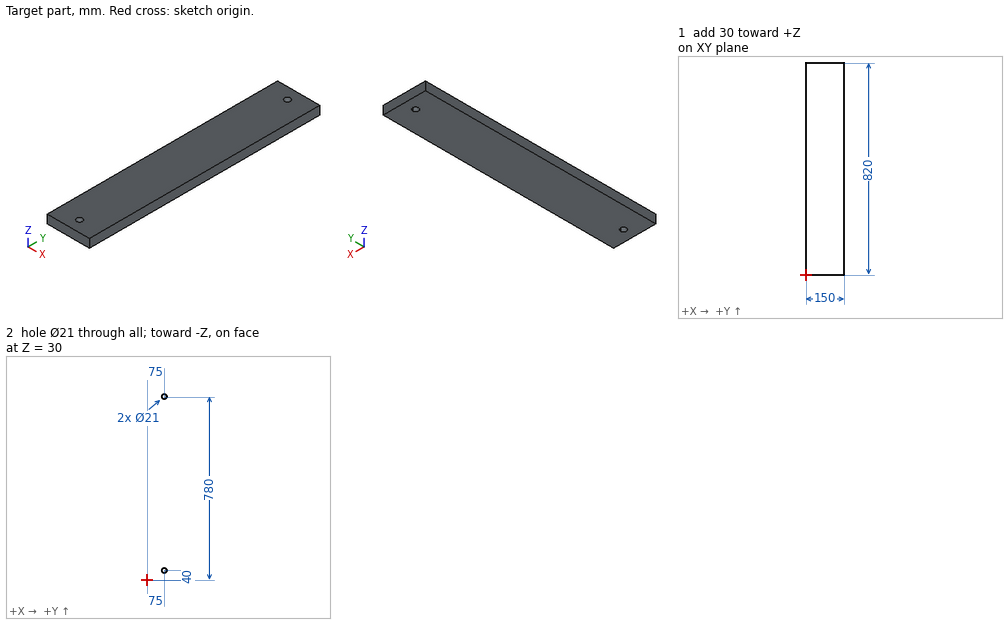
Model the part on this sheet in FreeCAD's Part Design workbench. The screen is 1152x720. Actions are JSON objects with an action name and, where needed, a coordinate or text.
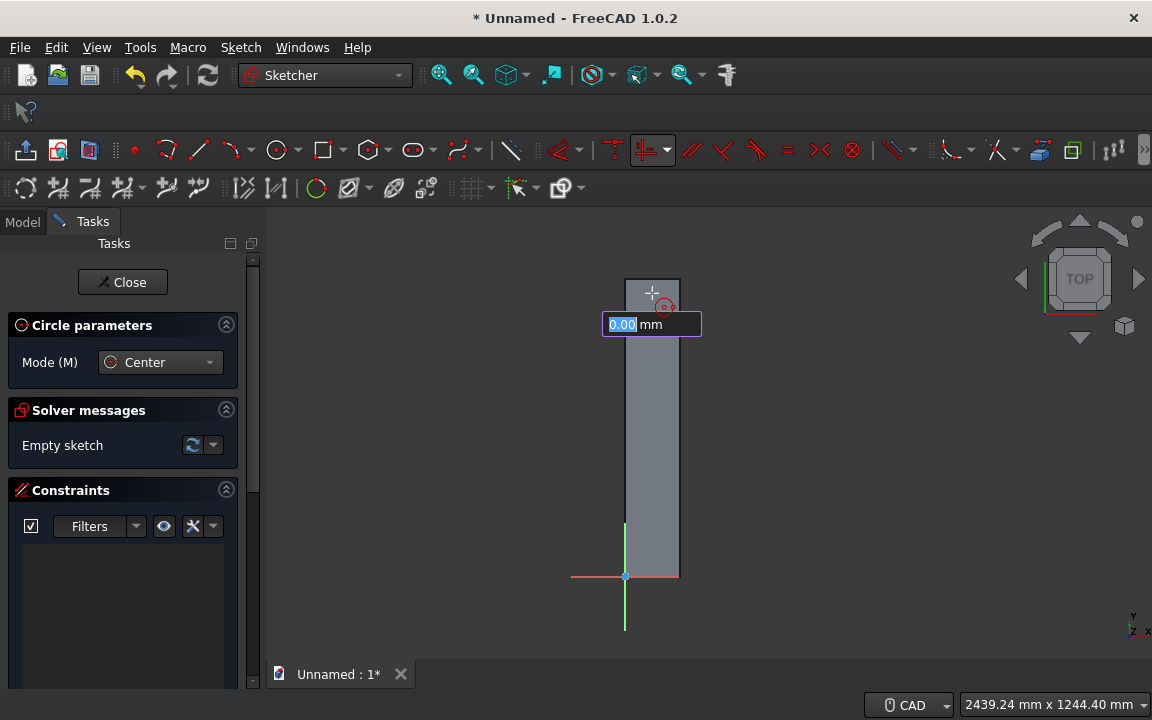
{"action": "scroll", "coordinate": [655, 291], "scroll_direction": "up", "scroll_amount": 8}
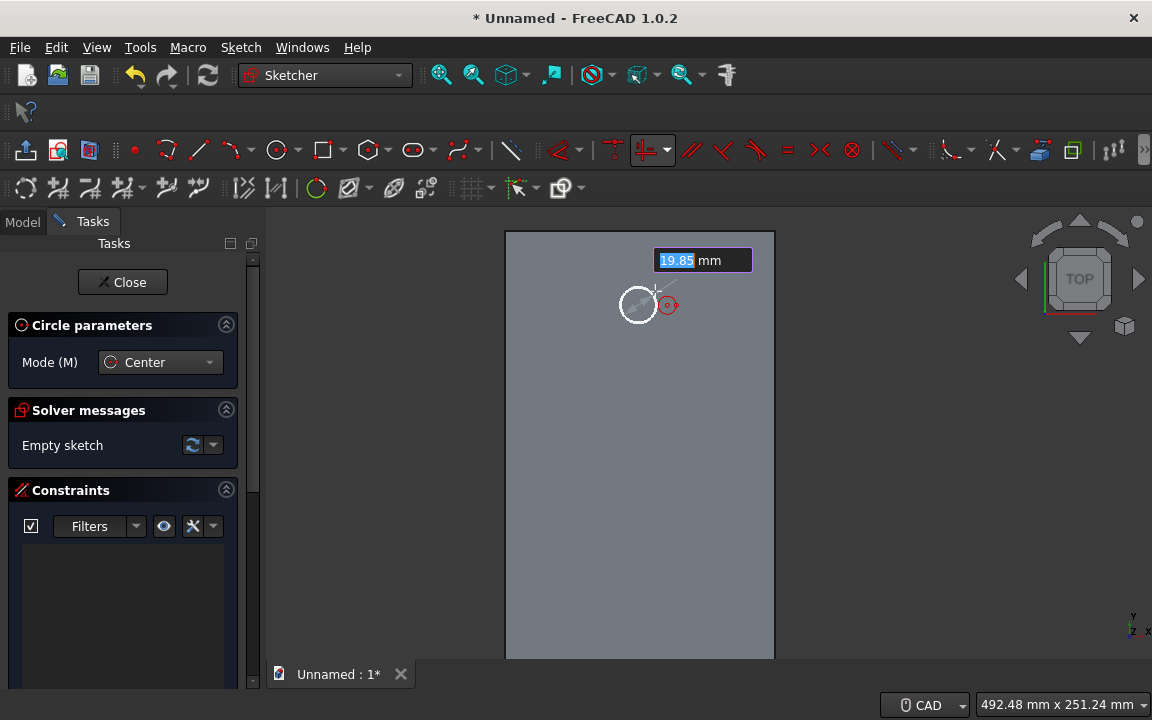
{"action": "left_click", "coordinate": [654, 289]}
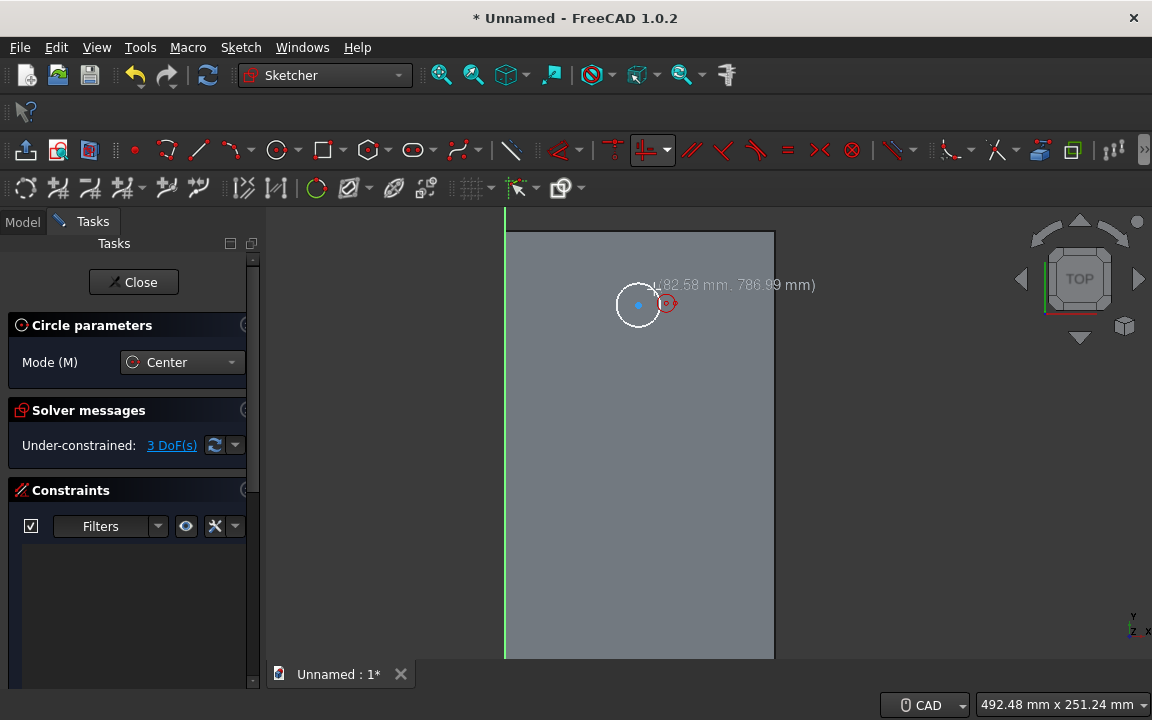
{"action": "scroll", "coordinate": [655, 291], "scroll_direction": "down", "scroll_amount": 8}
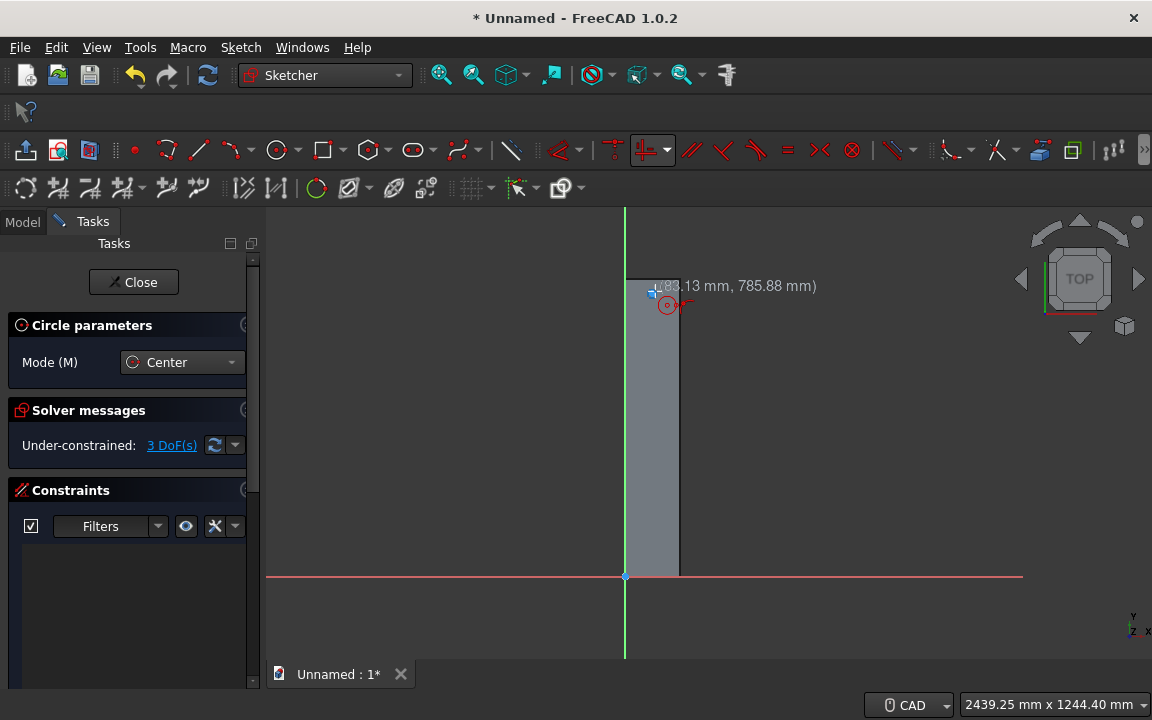
{"action": "scroll", "coordinate": [652, 562], "scroll_direction": "up", "scroll_amount": 9}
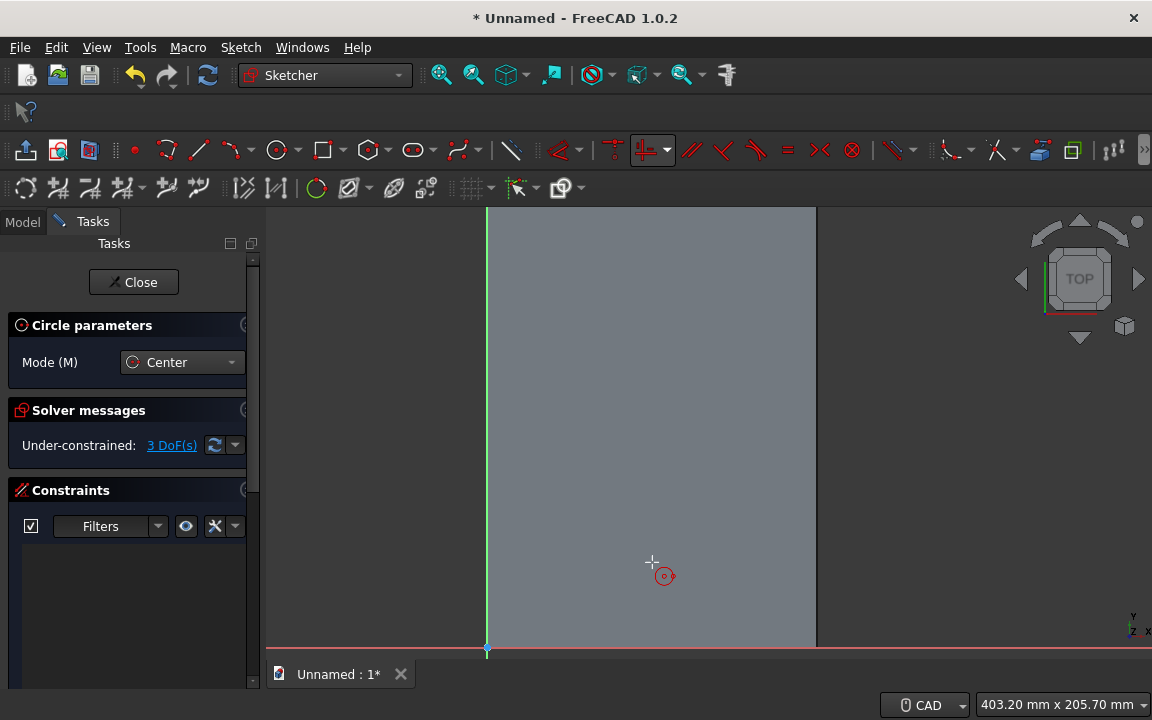
{"action": "scroll", "coordinate": [652, 563], "scroll_direction": "down", "scroll_amount": 9}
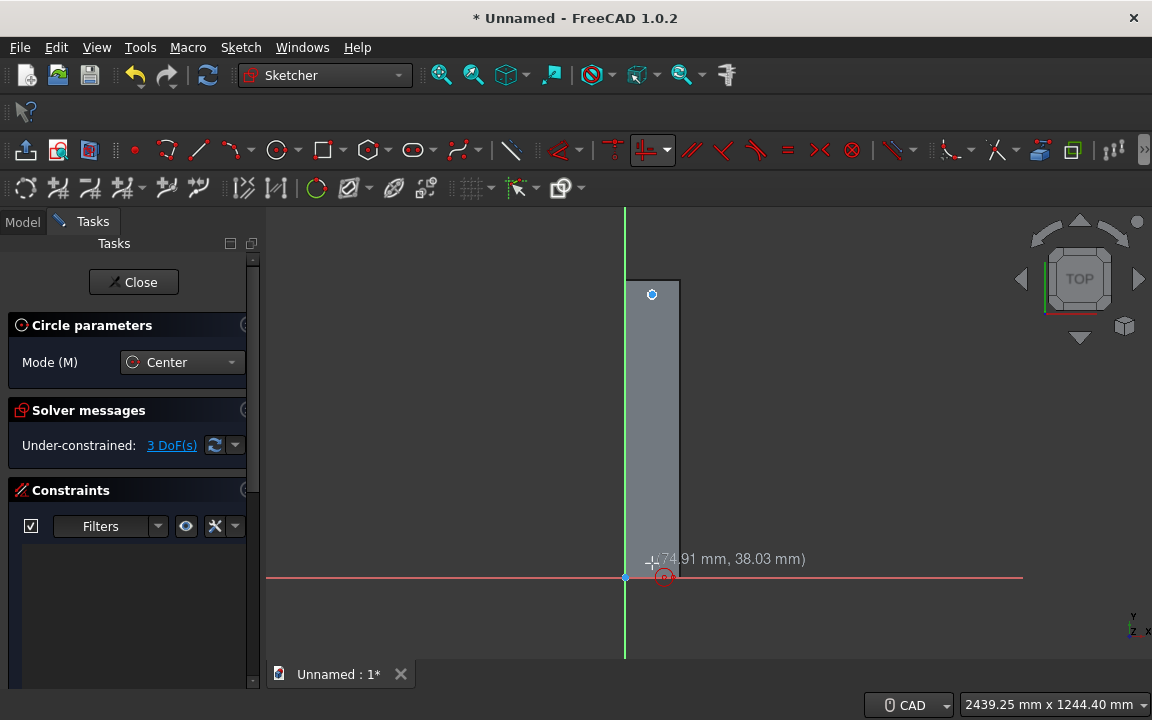
{"action": "left_click", "coordinate": [652, 563]}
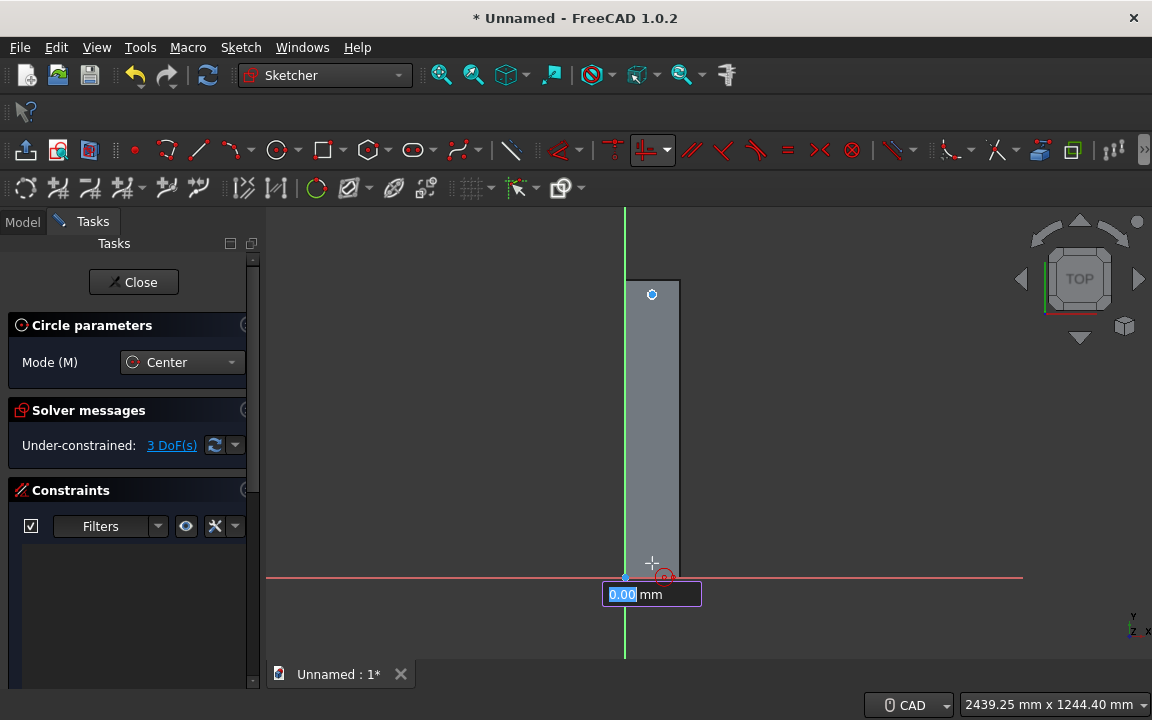
{"action": "scroll", "coordinate": [655, 560], "scroll_direction": "up", "scroll_amount": 8}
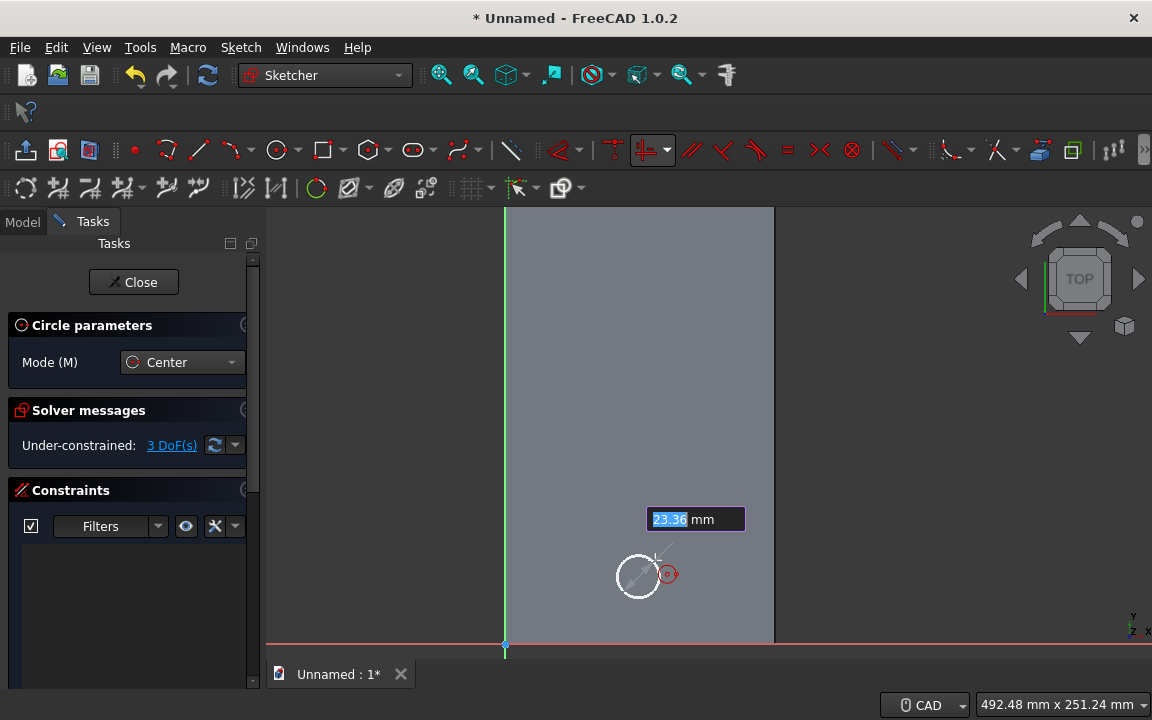
{"action": "left_click", "coordinate": [654, 559]}
{"action": "key", "text": "Escape"}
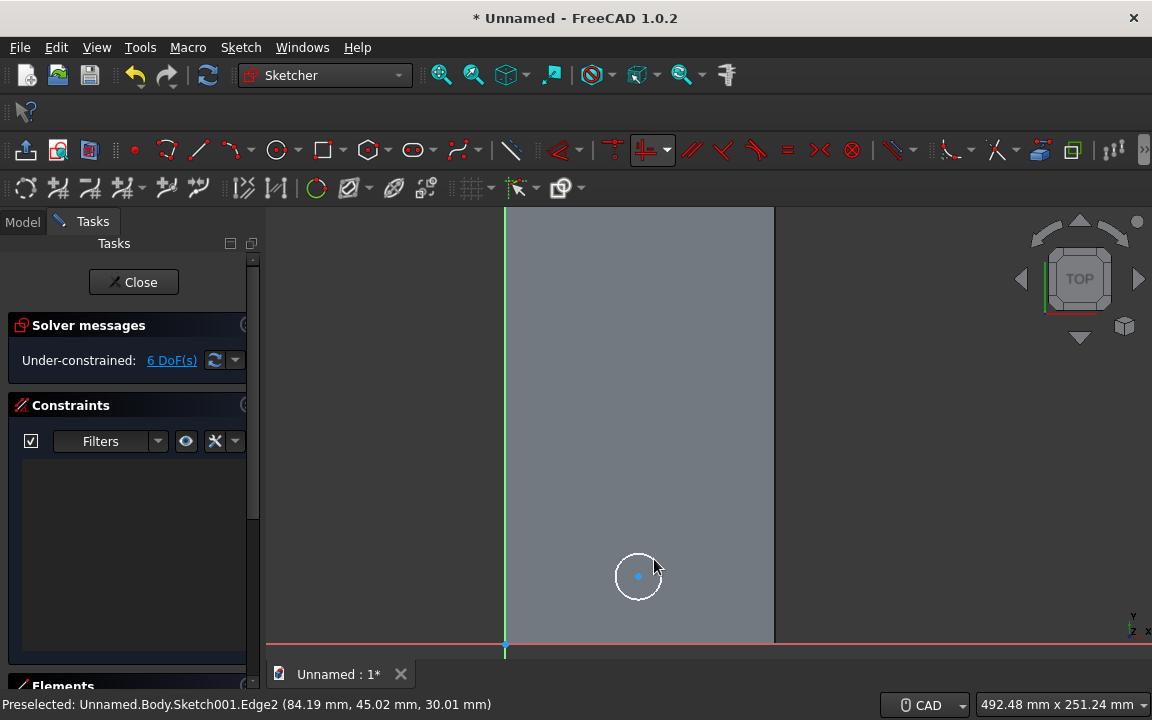
{"action": "scroll", "coordinate": [655, 559], "scroll_direction": "down", "scroll_amount": 8}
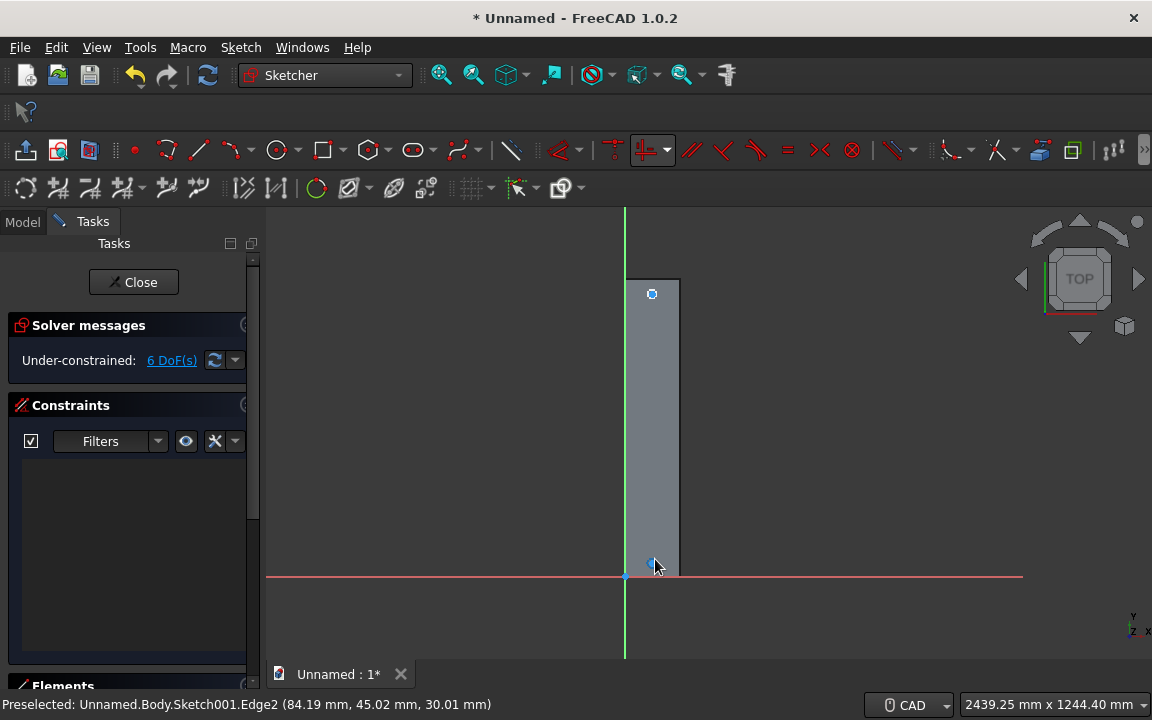
{"action": "scroll", "coordinate": [655, 291], "scroll_direction": "up", "scroll_amount": 6}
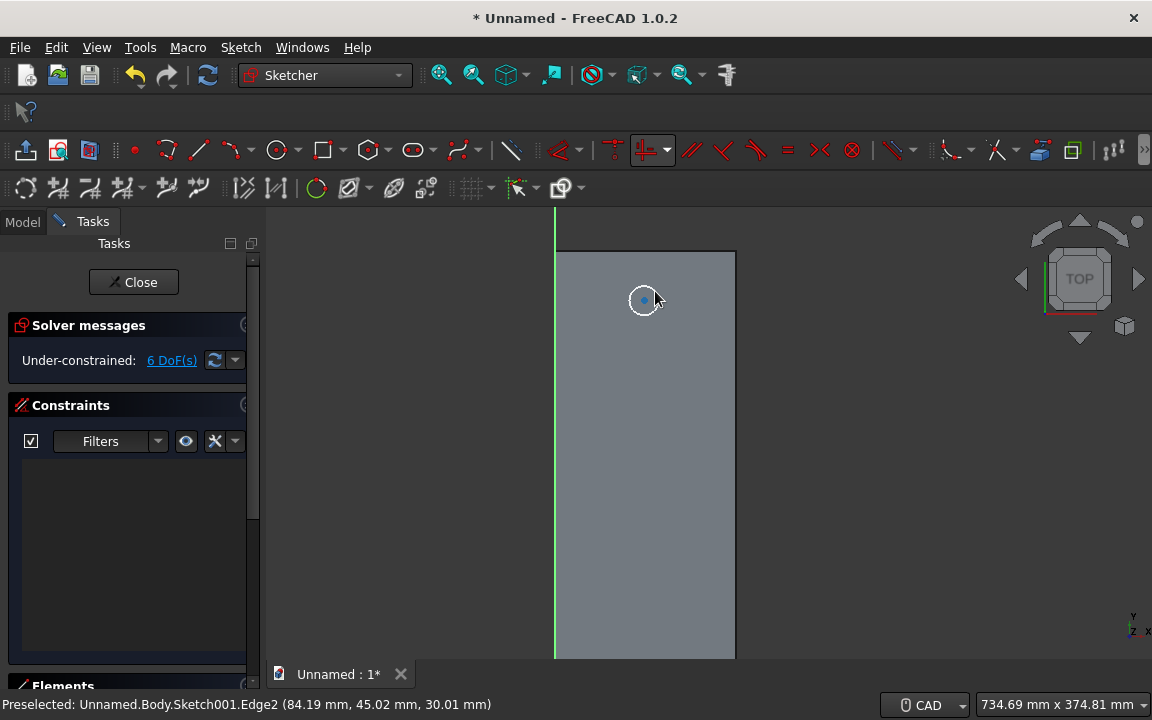
{"action": "left_click", "coordinate": [654, 290]}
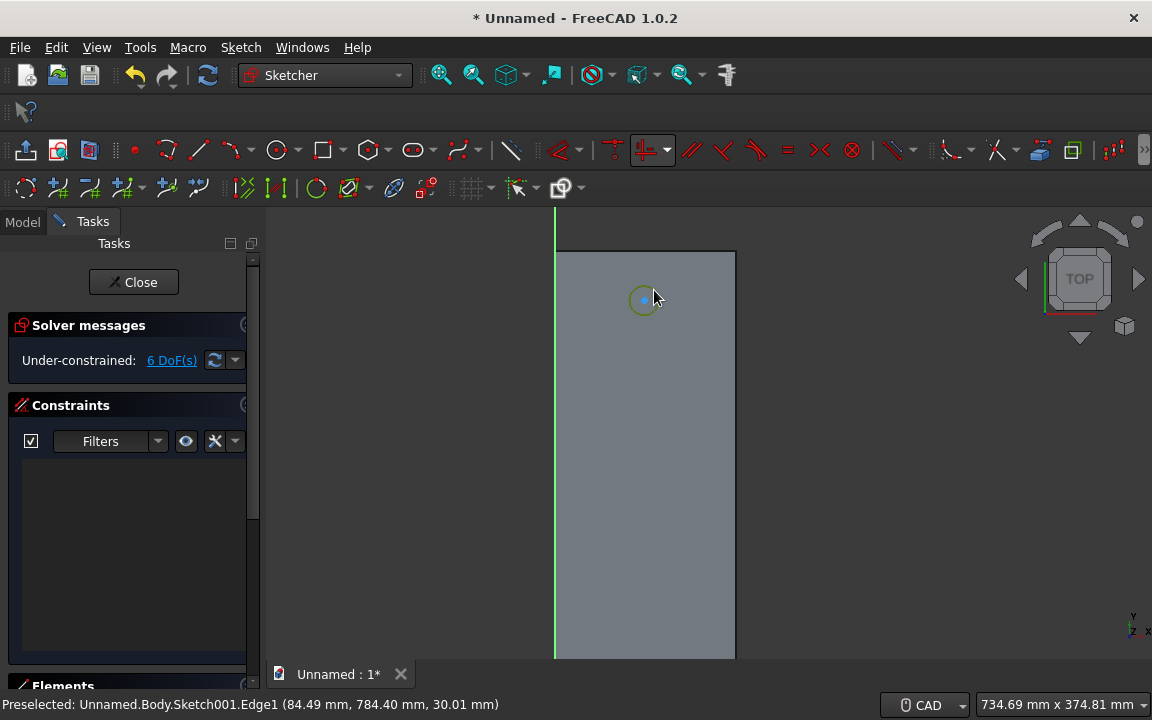
{"action": "scroll", "coordinate": [655, 291], "scroll_direction": "down", "scroll_amount": 6}